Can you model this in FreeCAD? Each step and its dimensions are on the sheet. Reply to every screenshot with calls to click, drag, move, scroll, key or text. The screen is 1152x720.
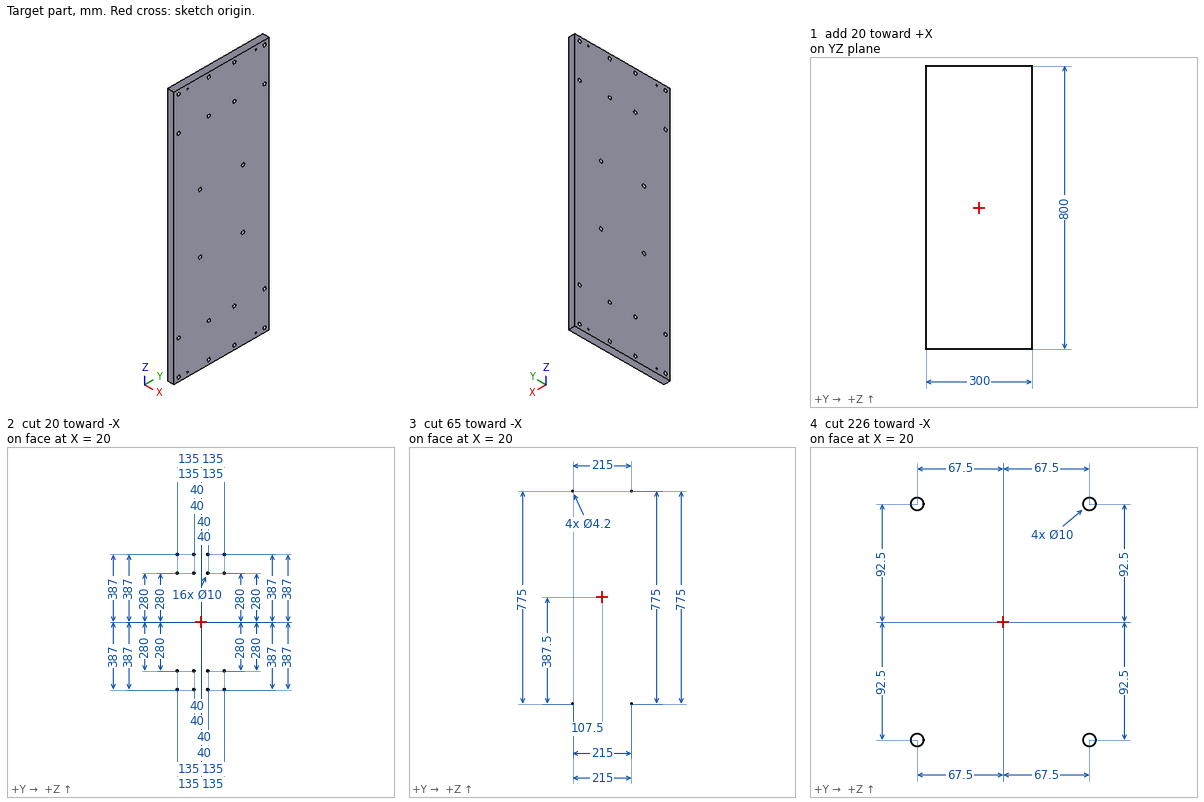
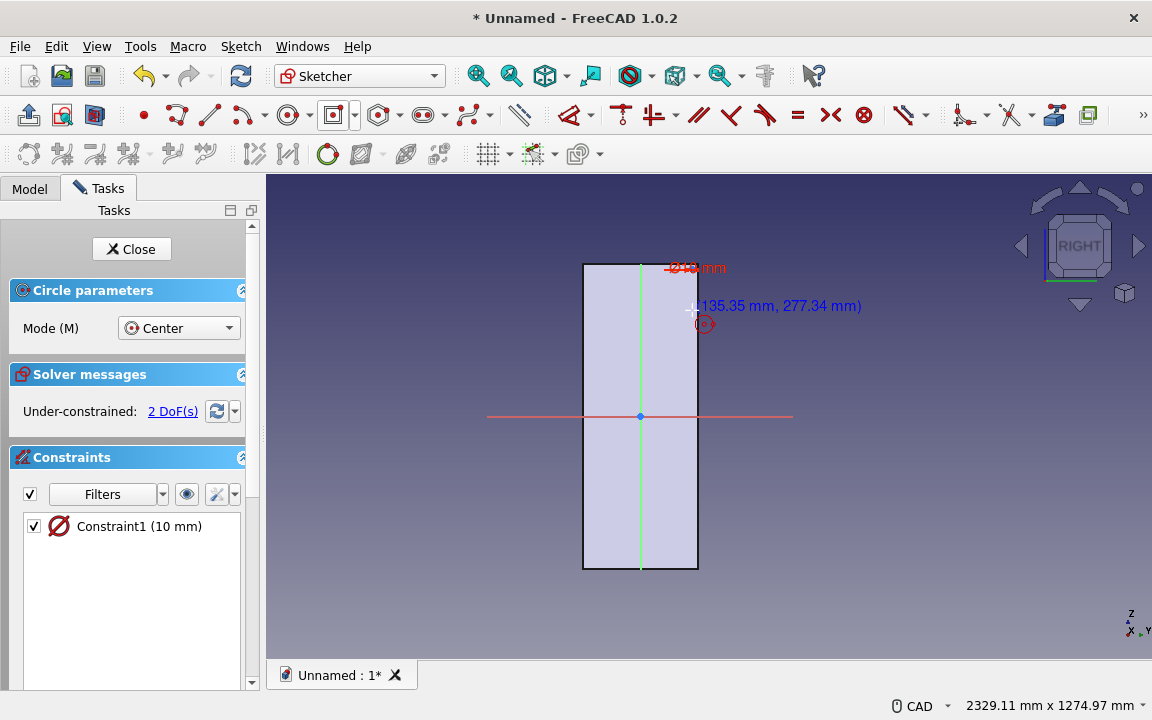
click(692, 310)
move(693, 309)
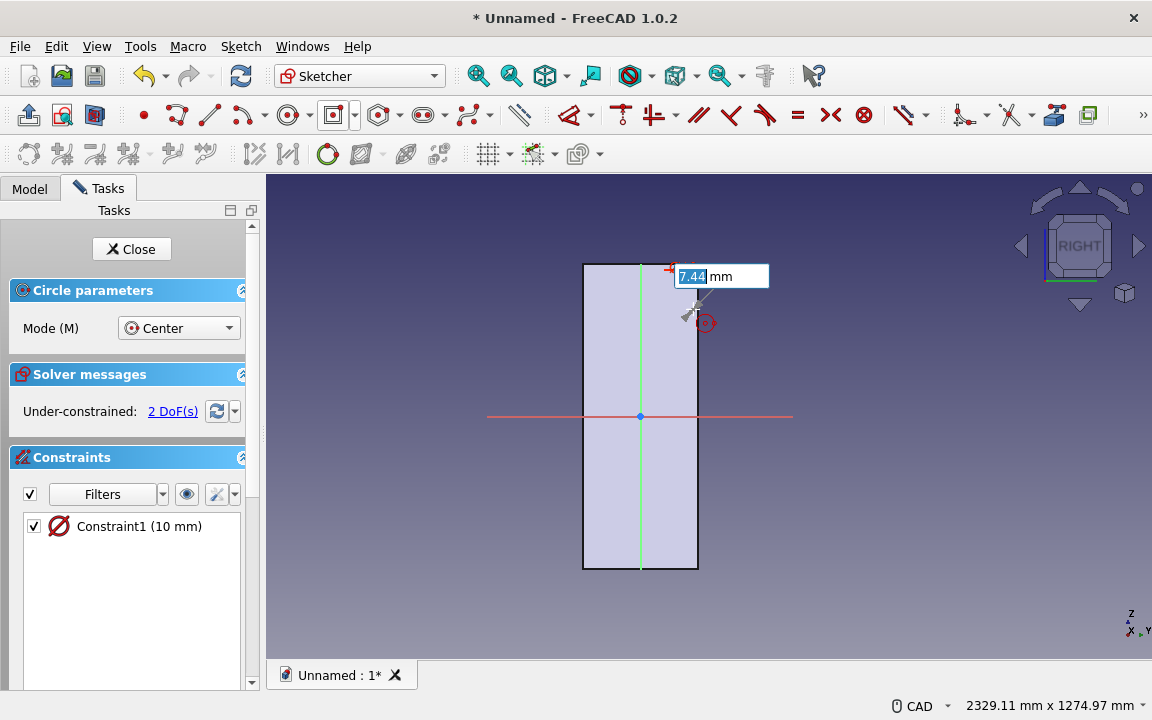
text(10)
key(Return)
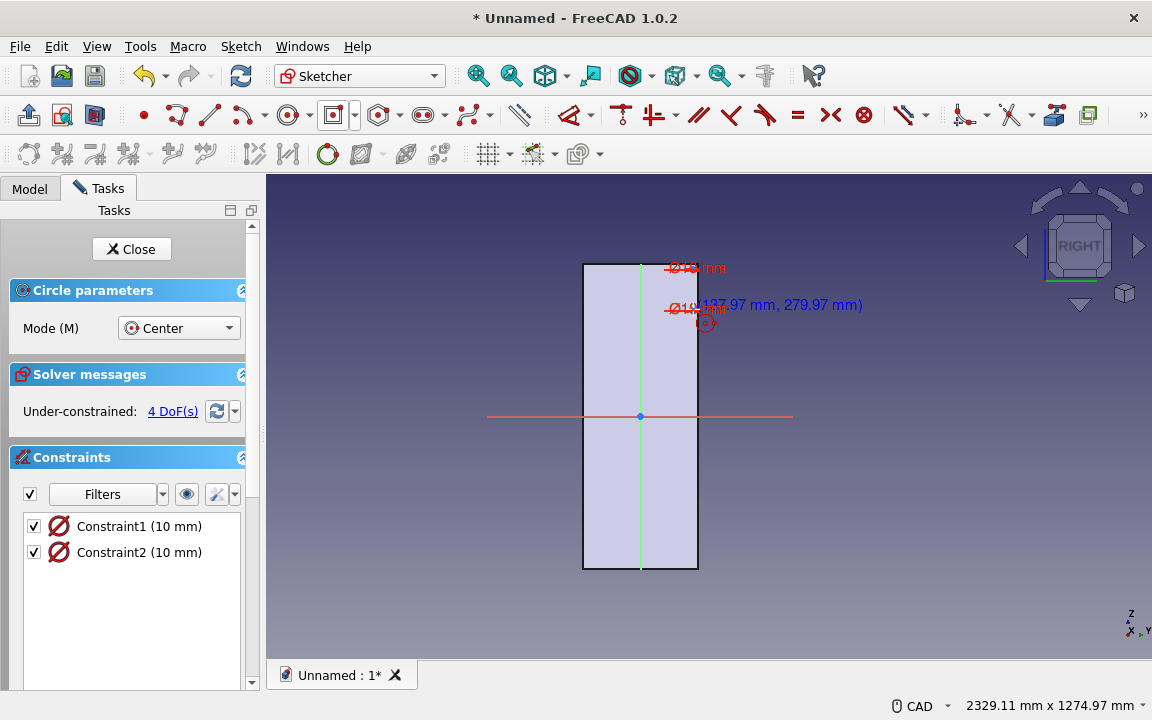
scroll(656, 310, up, 13)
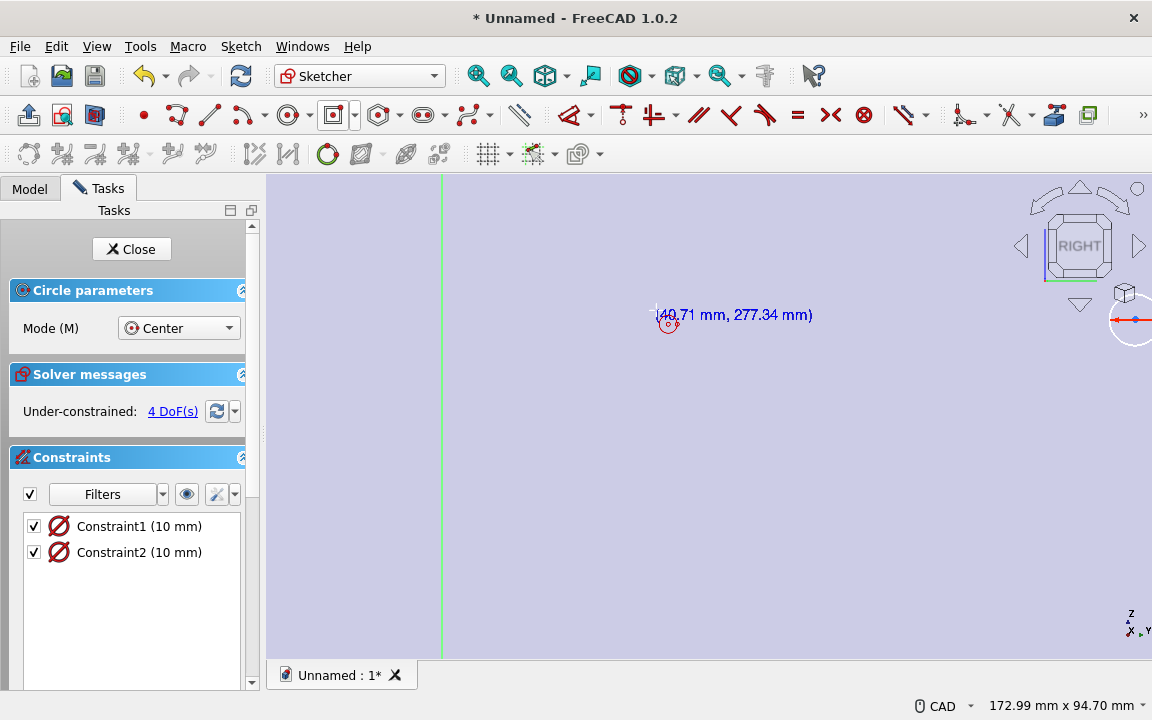
scroll(656, 310, down, 13)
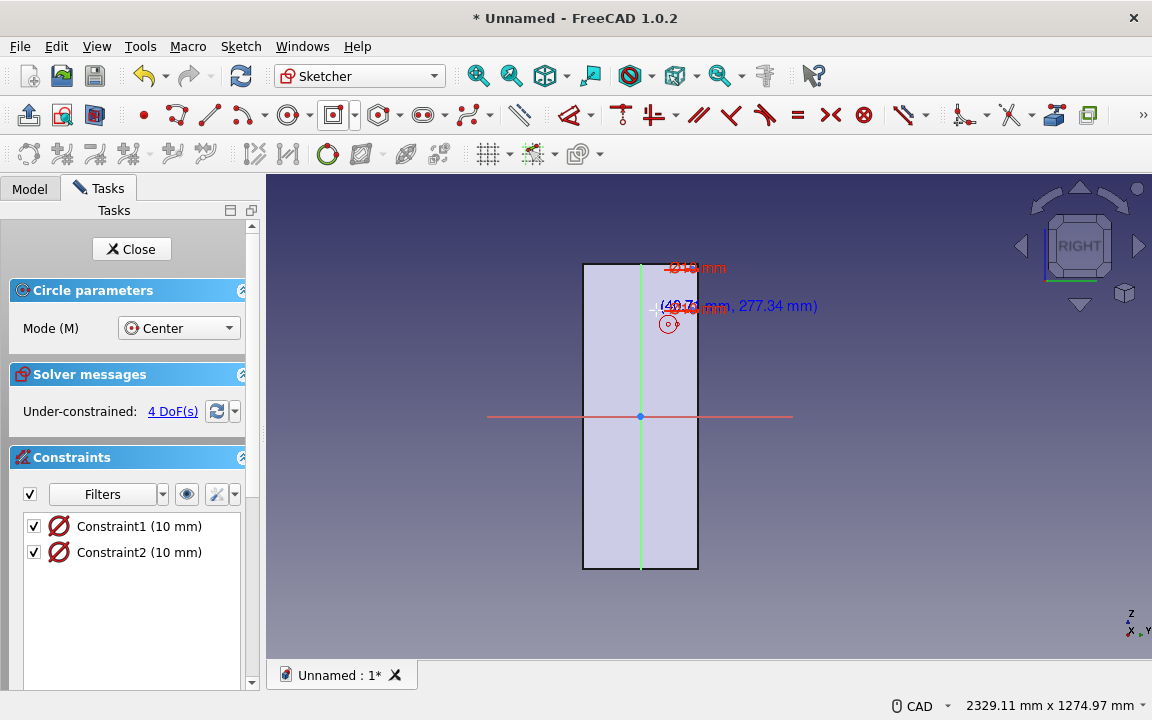
click(656, 310)
move(657, 309)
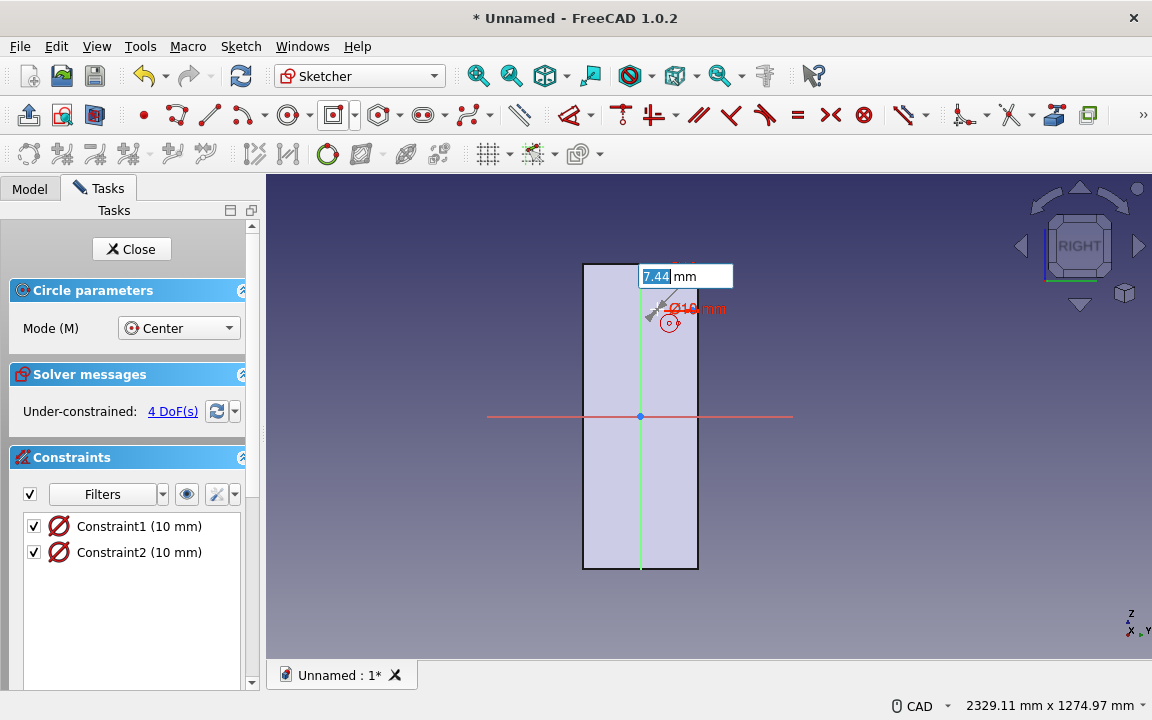
text(10)
key(Return)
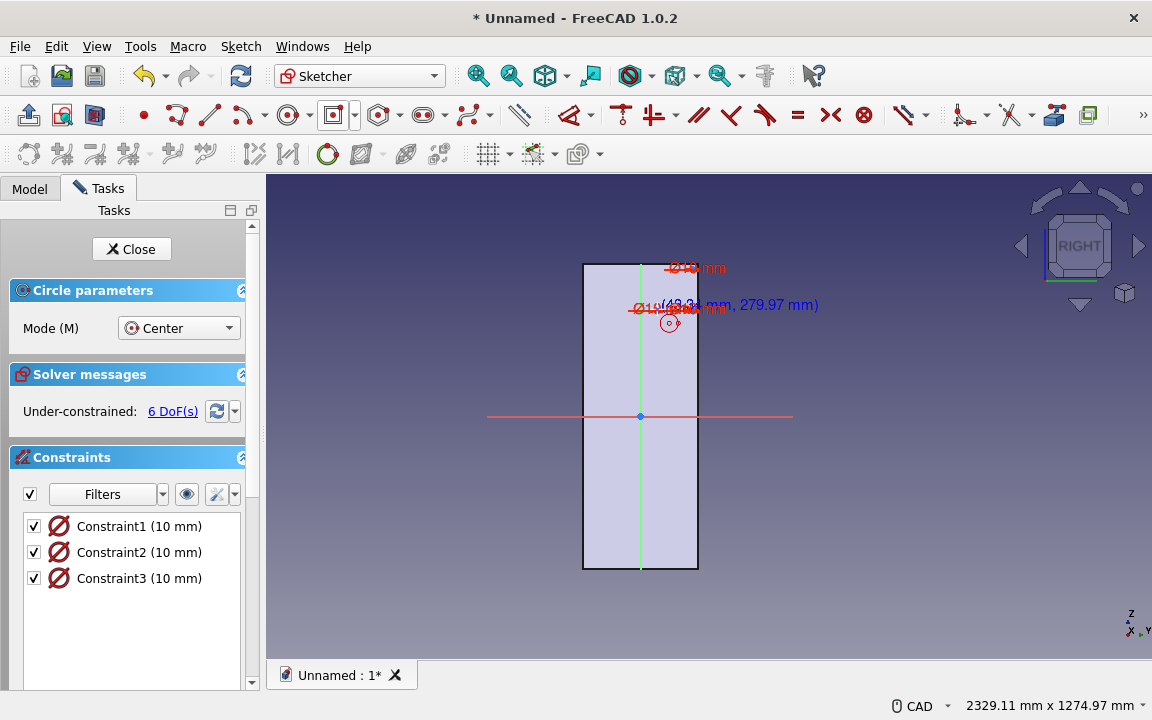
scroll(656, 269, up, 13)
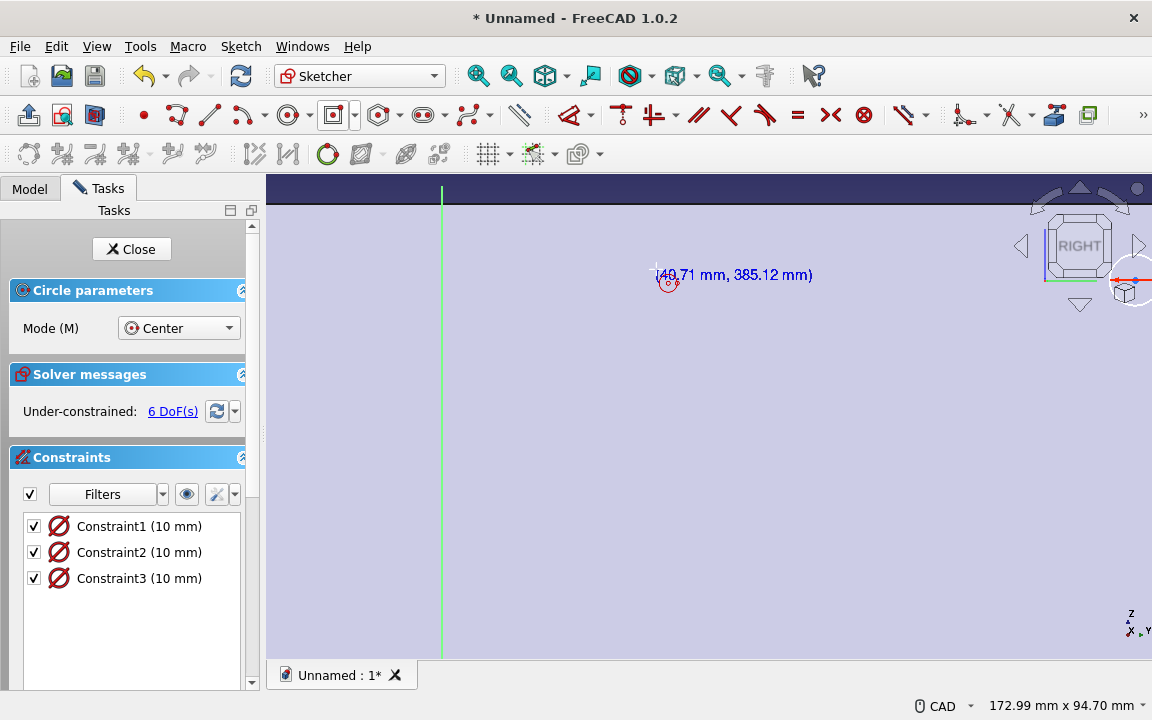
scroll(656, 269, down, 13)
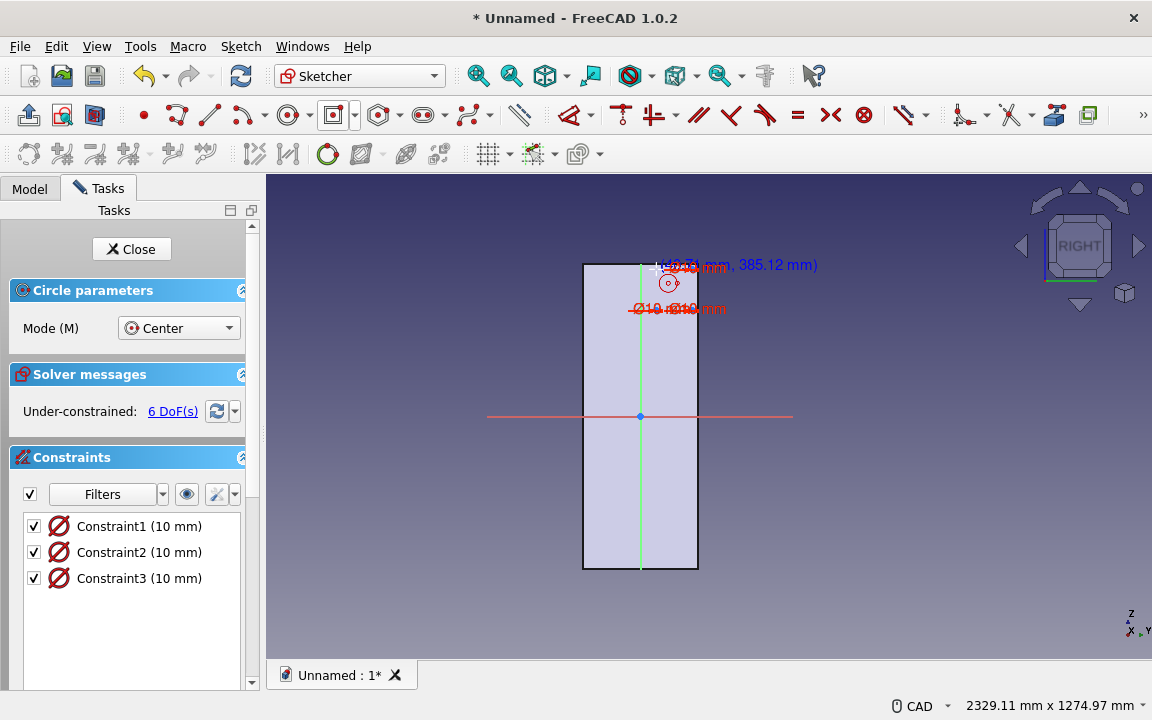
click(656, 269)
move(657, 268)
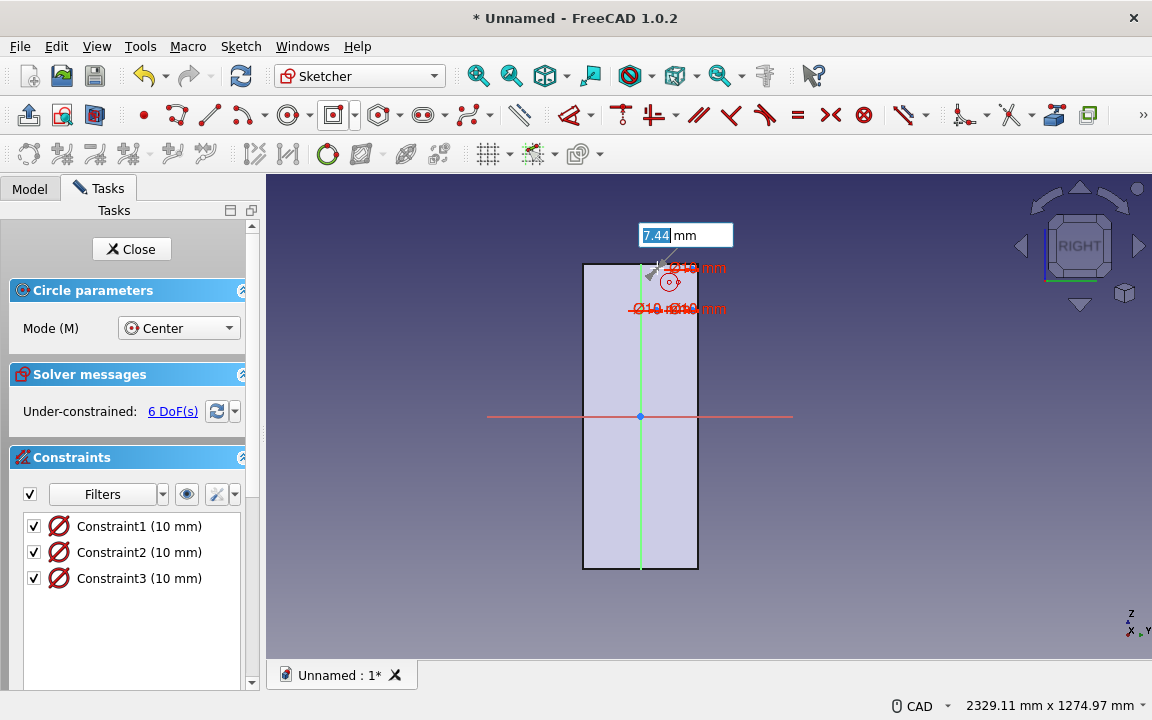
text(10)
key(Return)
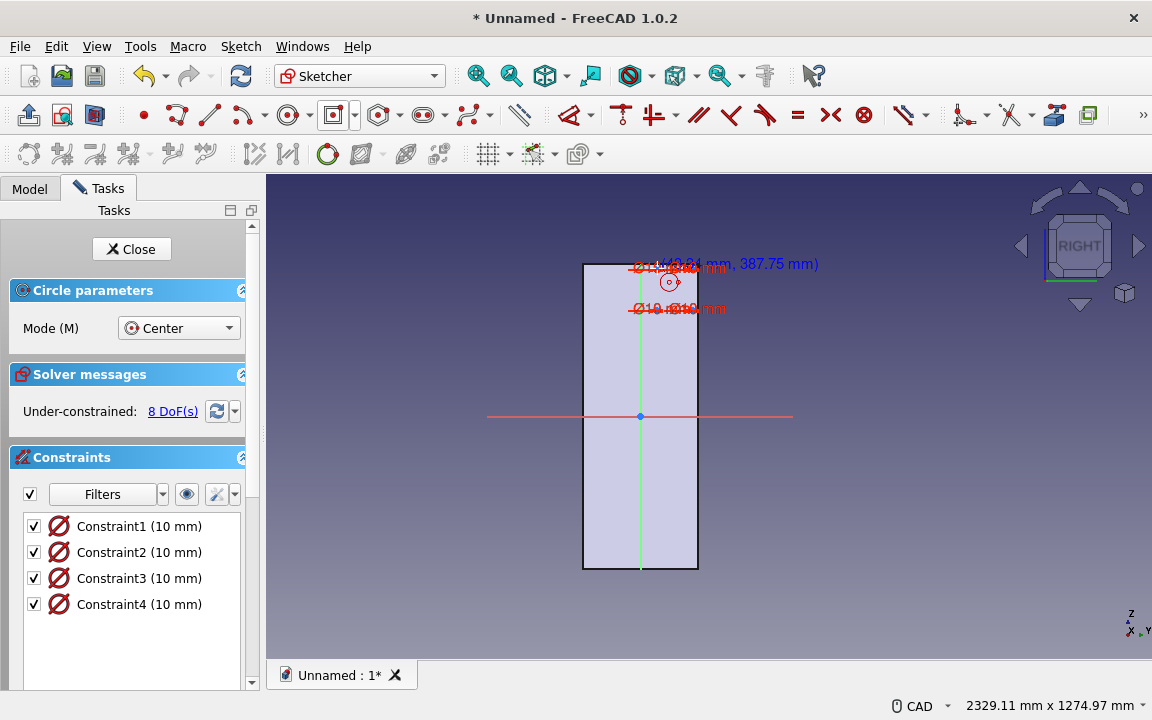
scroll(625, 310, up, 13)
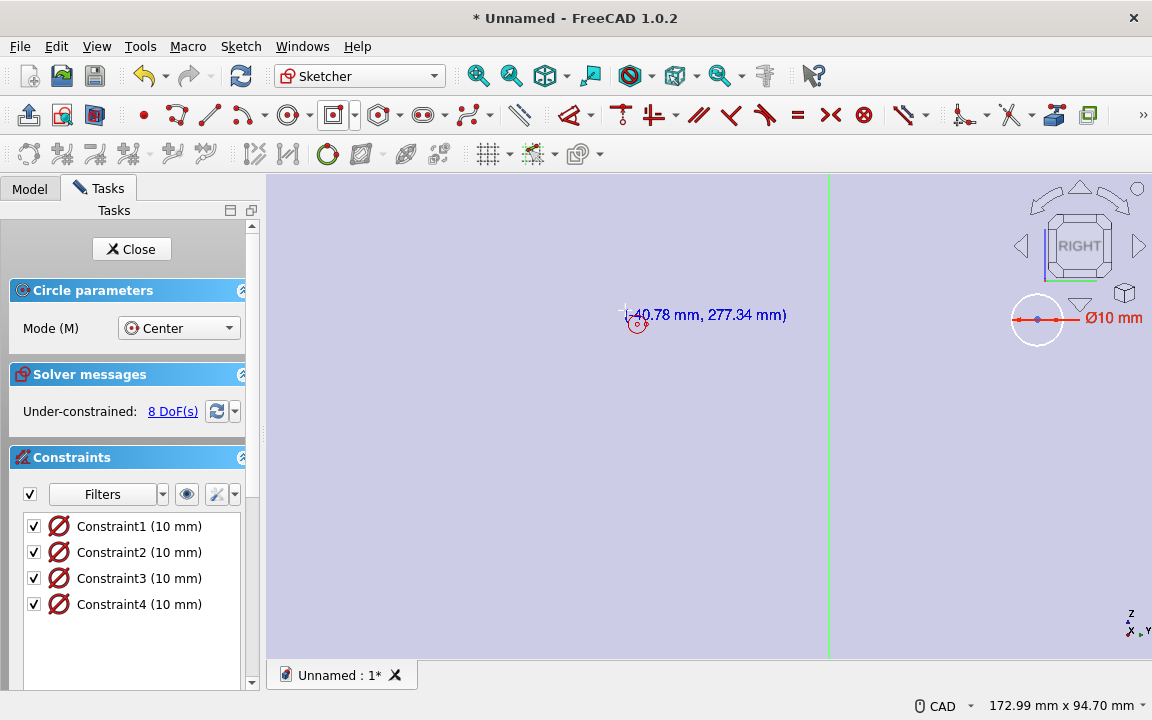
scroll(625, 310, down, 13)